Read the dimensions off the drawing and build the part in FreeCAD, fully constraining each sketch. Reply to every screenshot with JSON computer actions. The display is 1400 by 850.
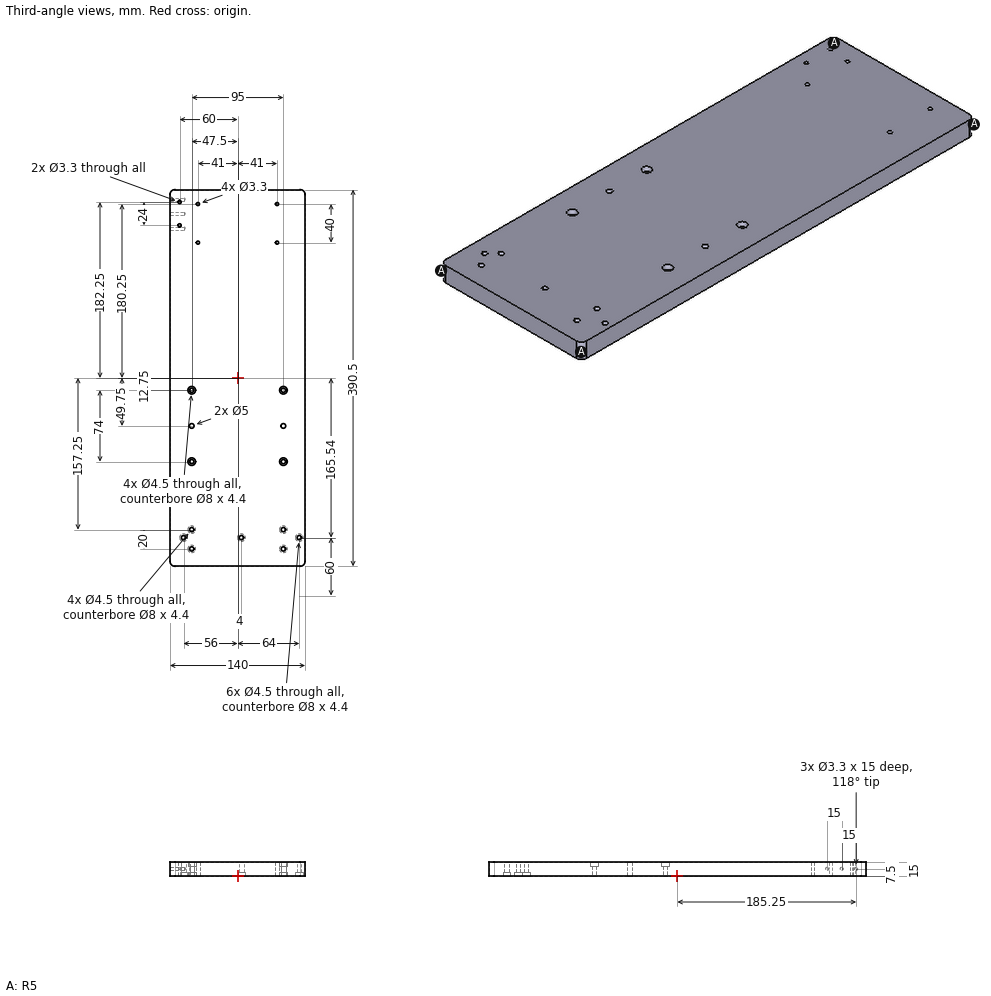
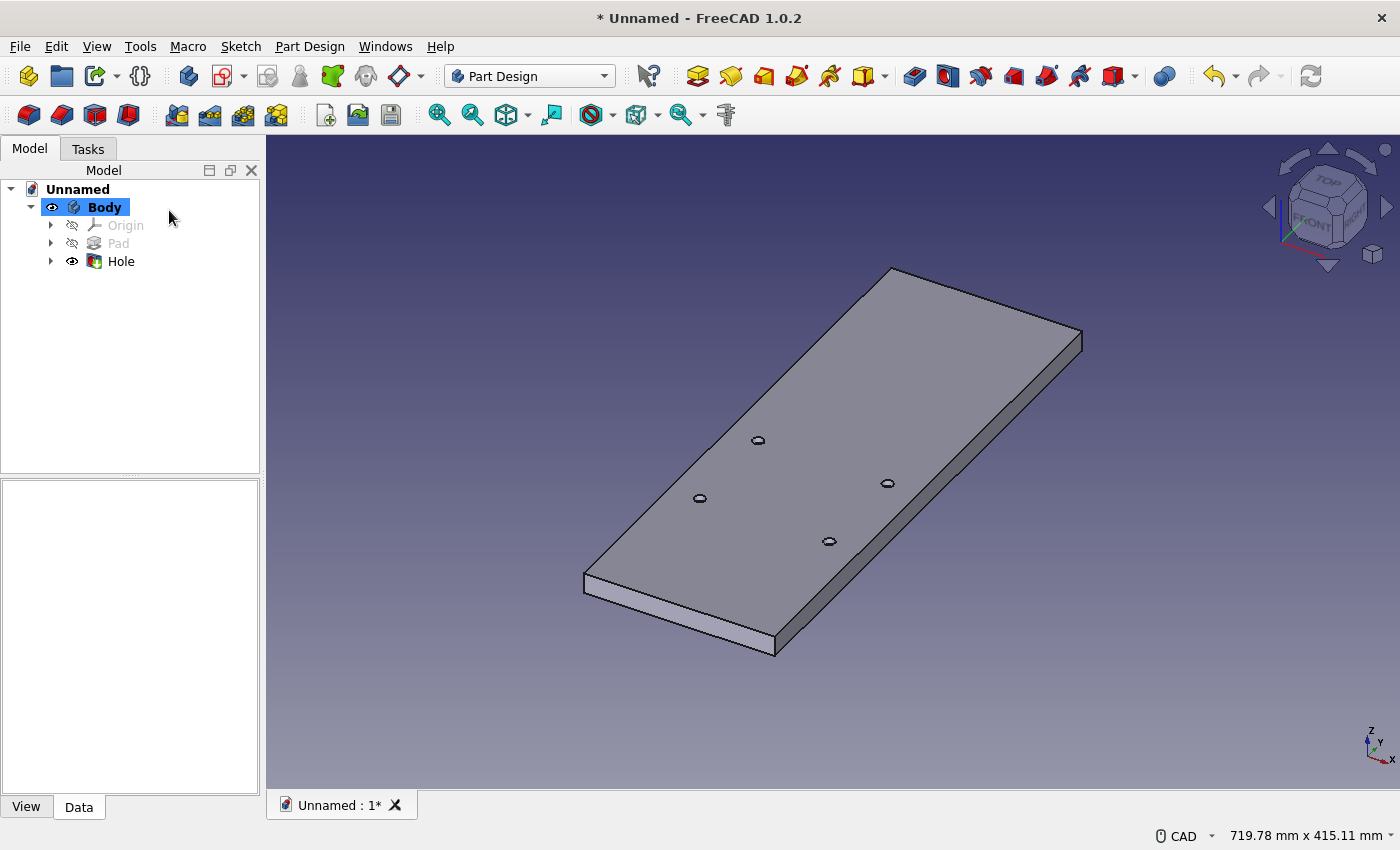
{"action": "left_click", "coordinate": [921, 364]}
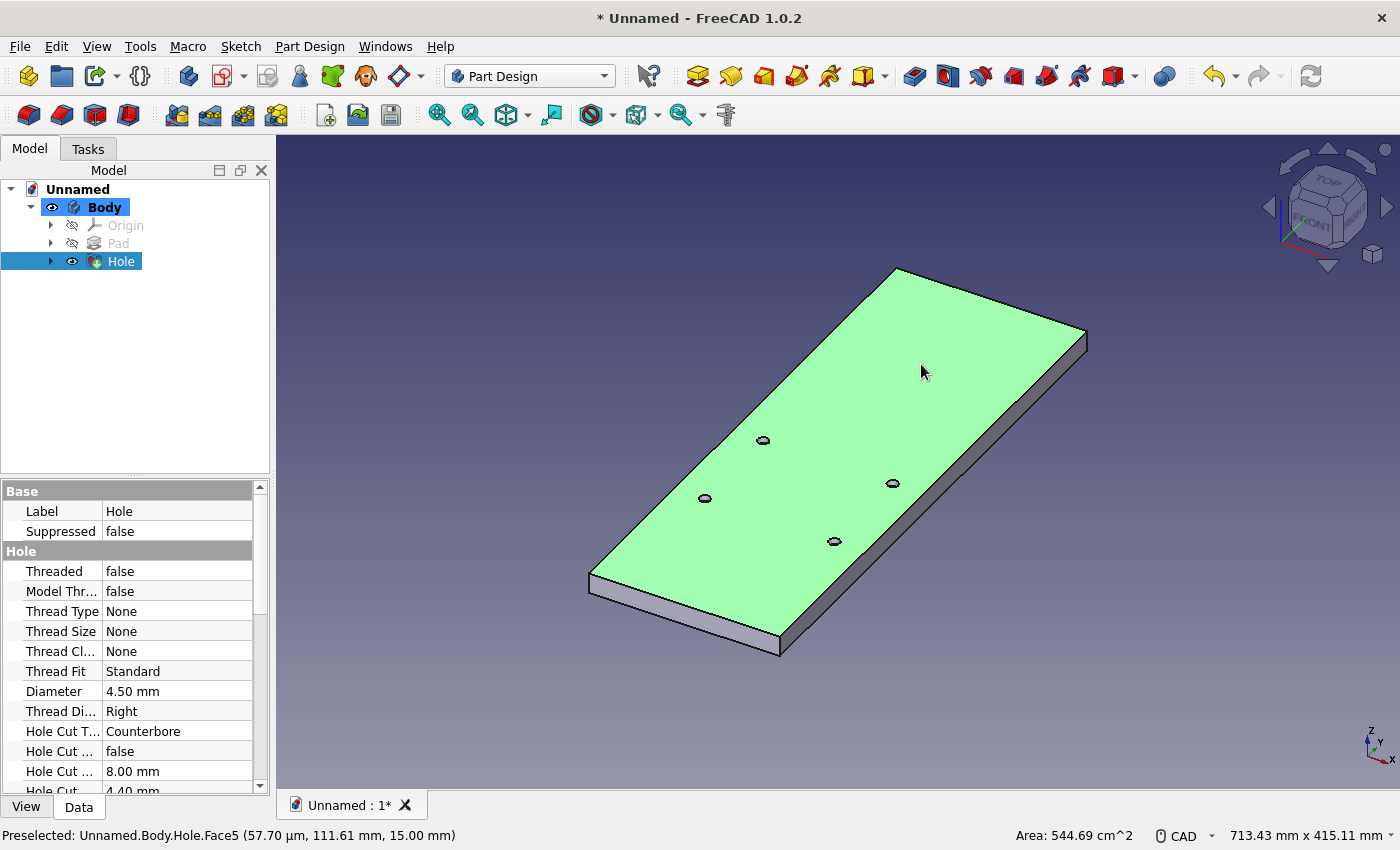
{"action": "left_click", "coordinate": [222, 76]}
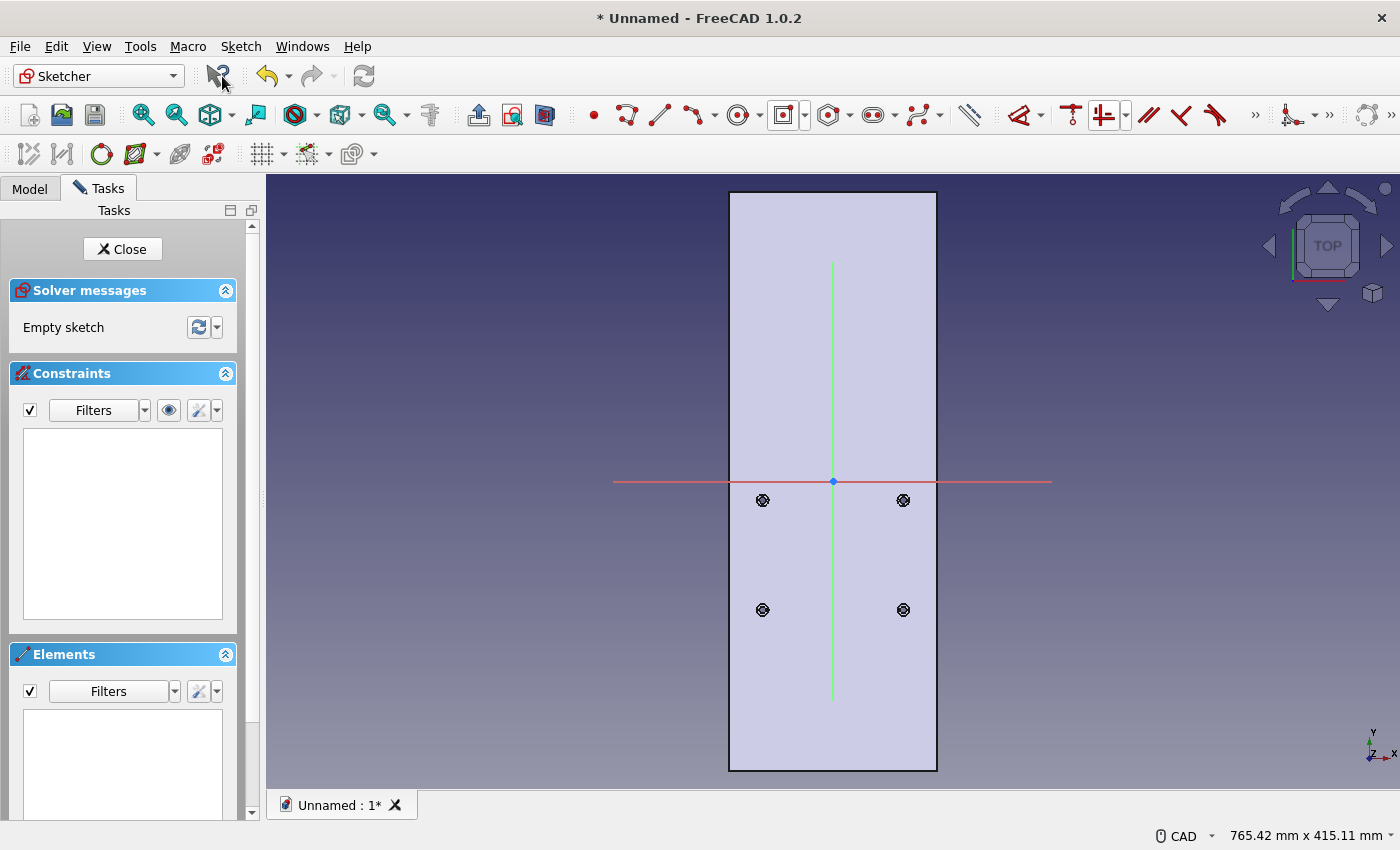
{"action": "scroll", "coordinate": [850, 530], "scroll_direction": "up", "scroll_amount": 8}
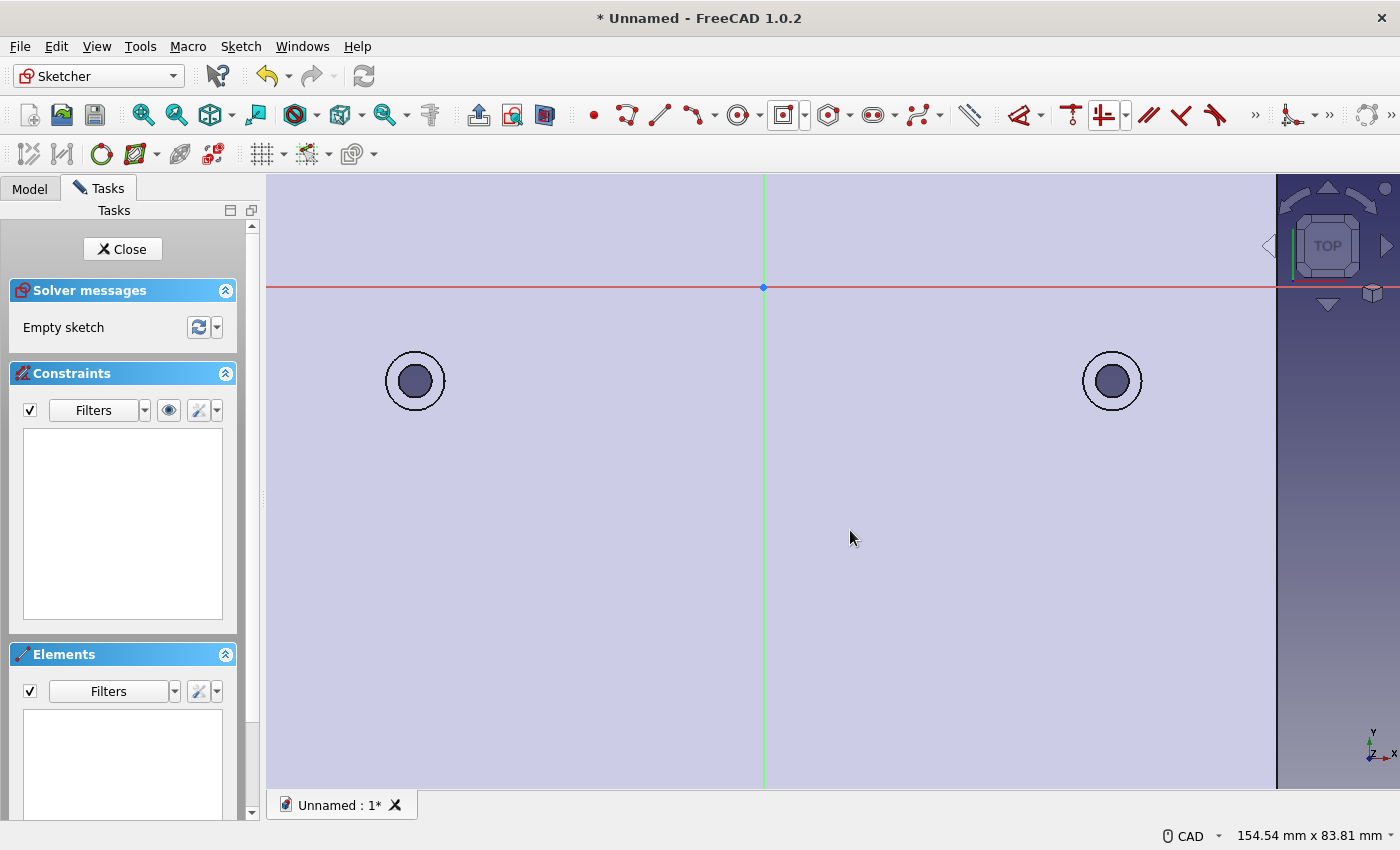
{"action": "left_click", "coordinate": [738, 116]}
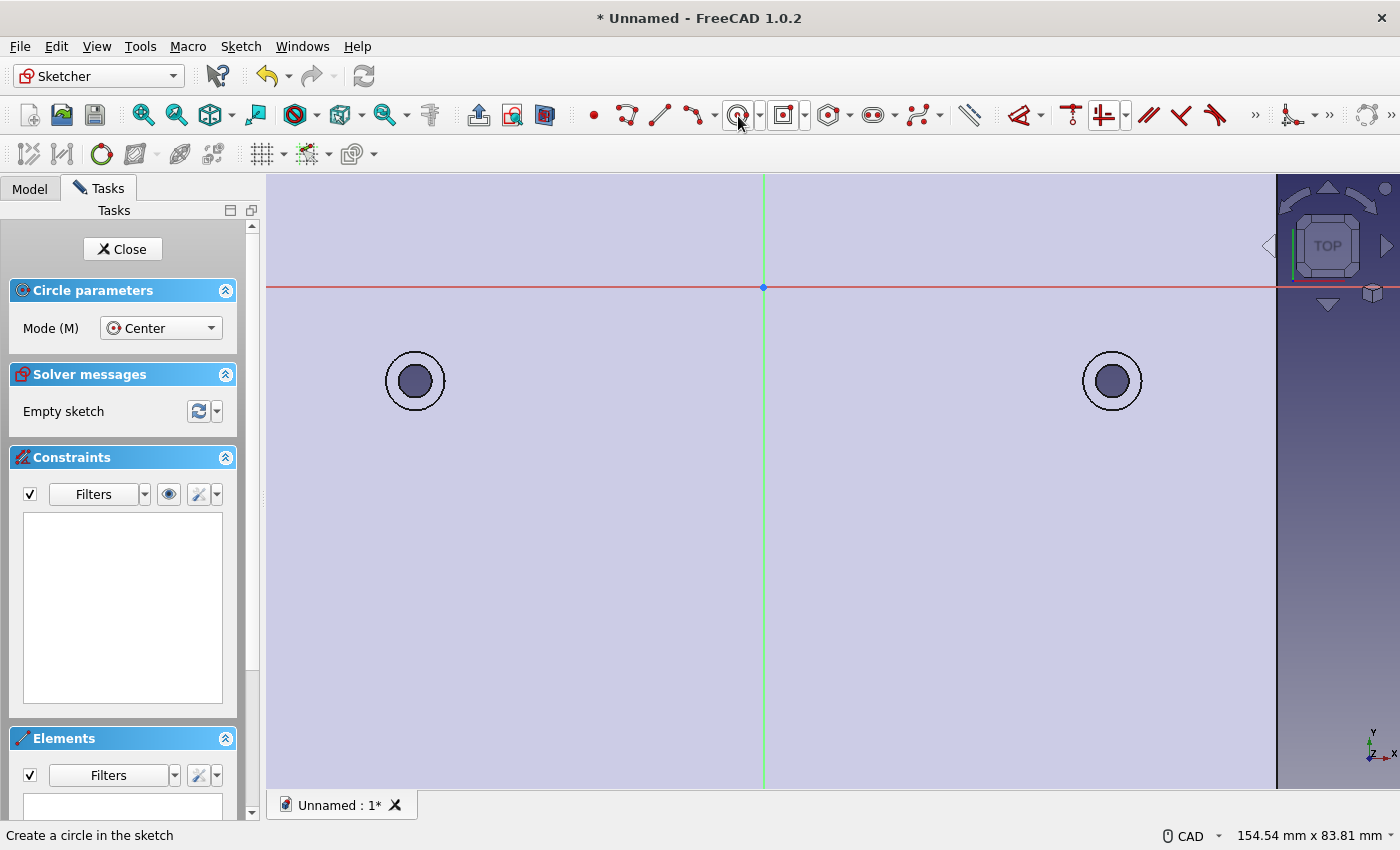
{"action": "scroll", "coordinate": [415, 653], "scroll_direction": "up", "scroll_amount": 2}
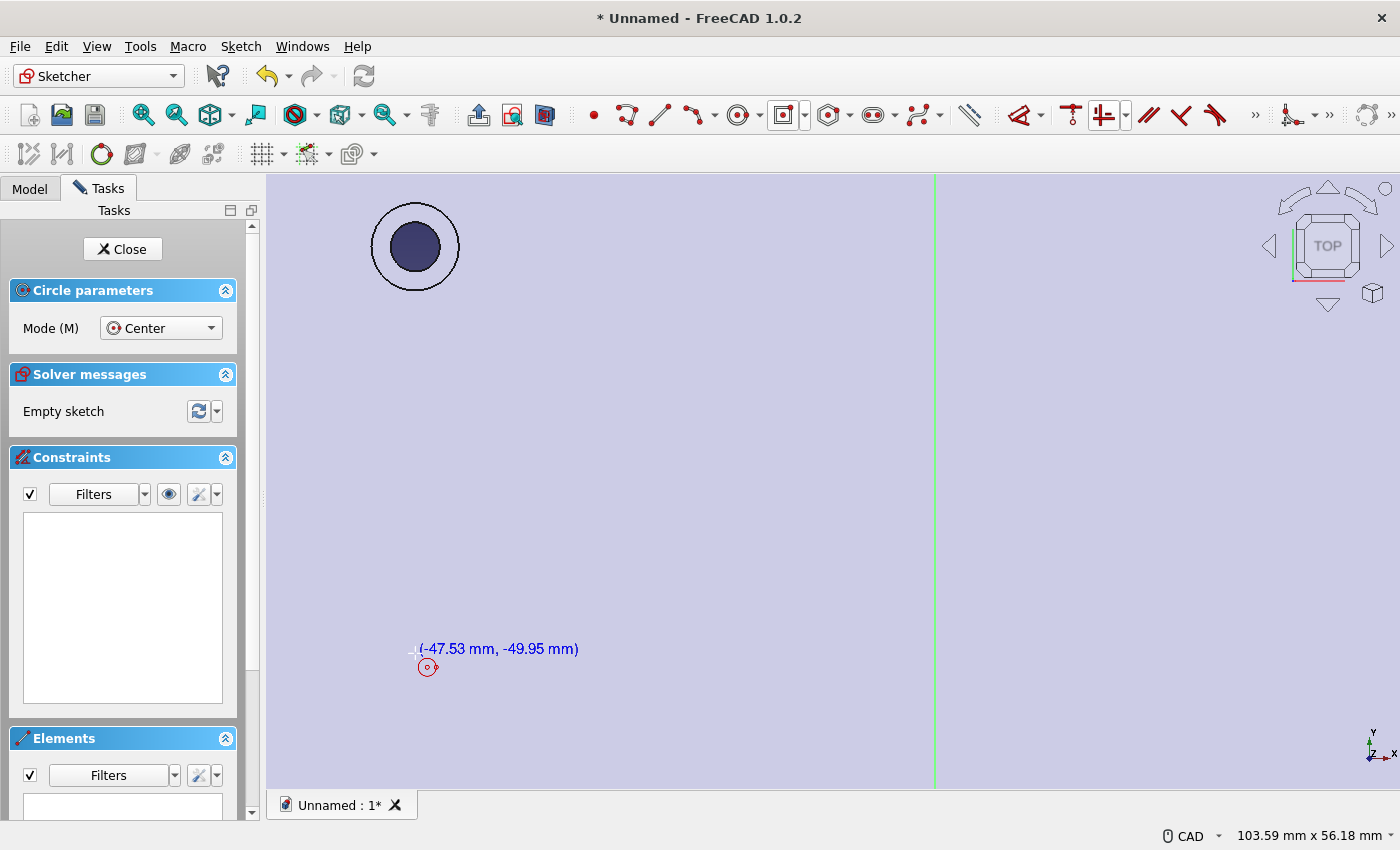
{"action": "left_click", "coordinate": [415, 652]}
{"action": "mouse_move", "coordinate": [435, 633]}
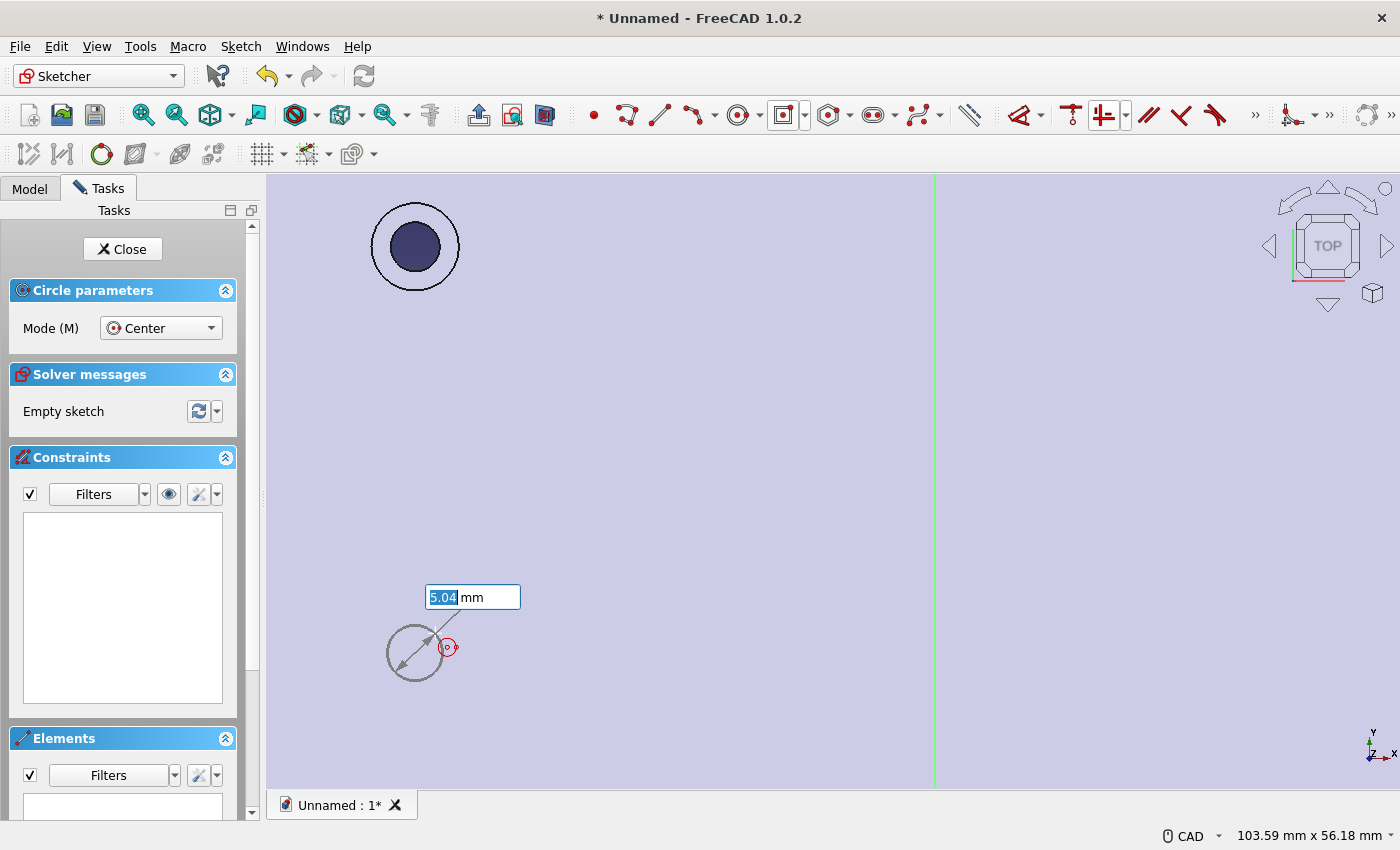
{"action": "type", "text": "5"}
{"action": "key", "text": "Return"}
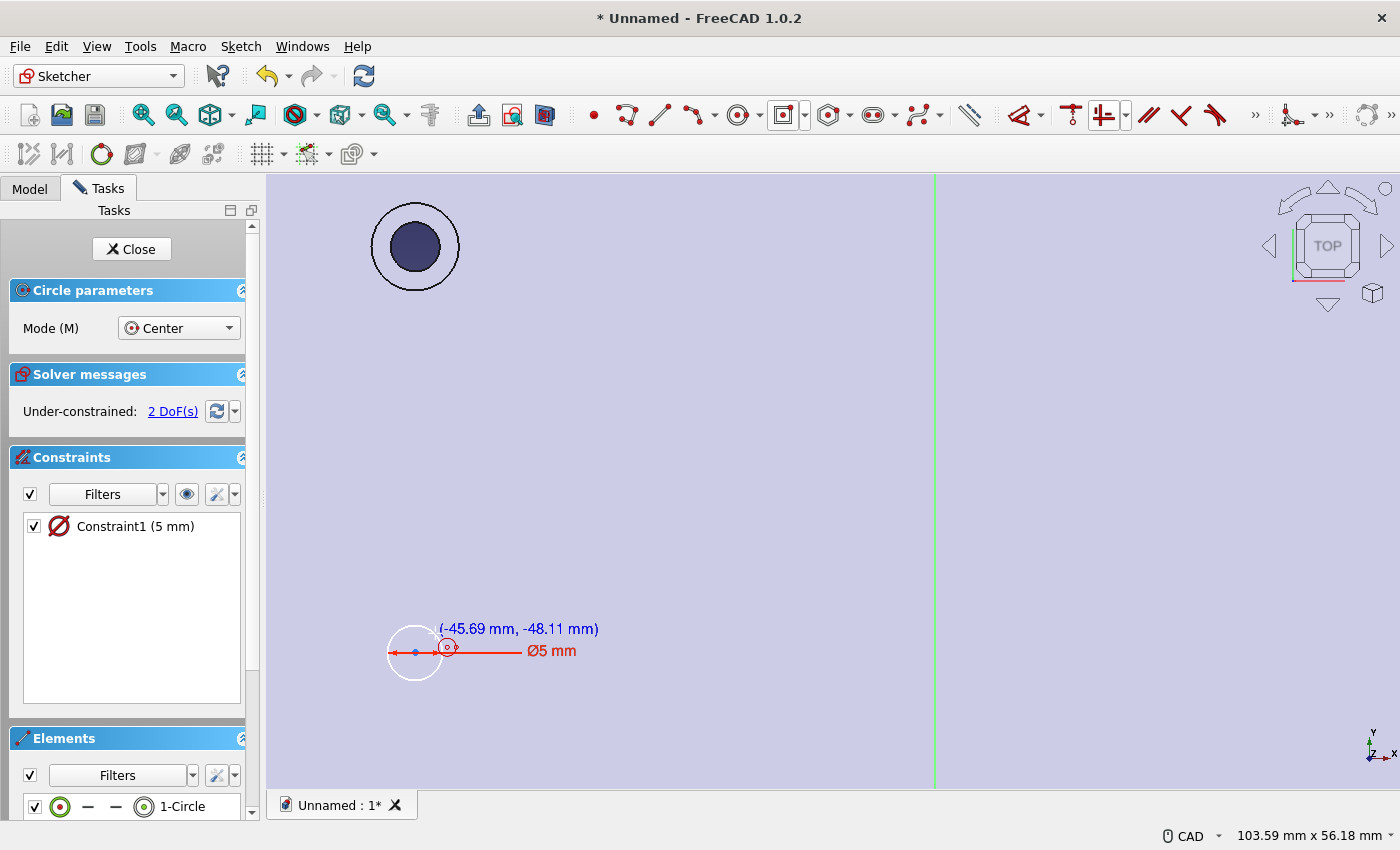
{"action": "scroll", "coordinate": [417, 661], "scroll_direction": "down", "scroll_amount": 2}